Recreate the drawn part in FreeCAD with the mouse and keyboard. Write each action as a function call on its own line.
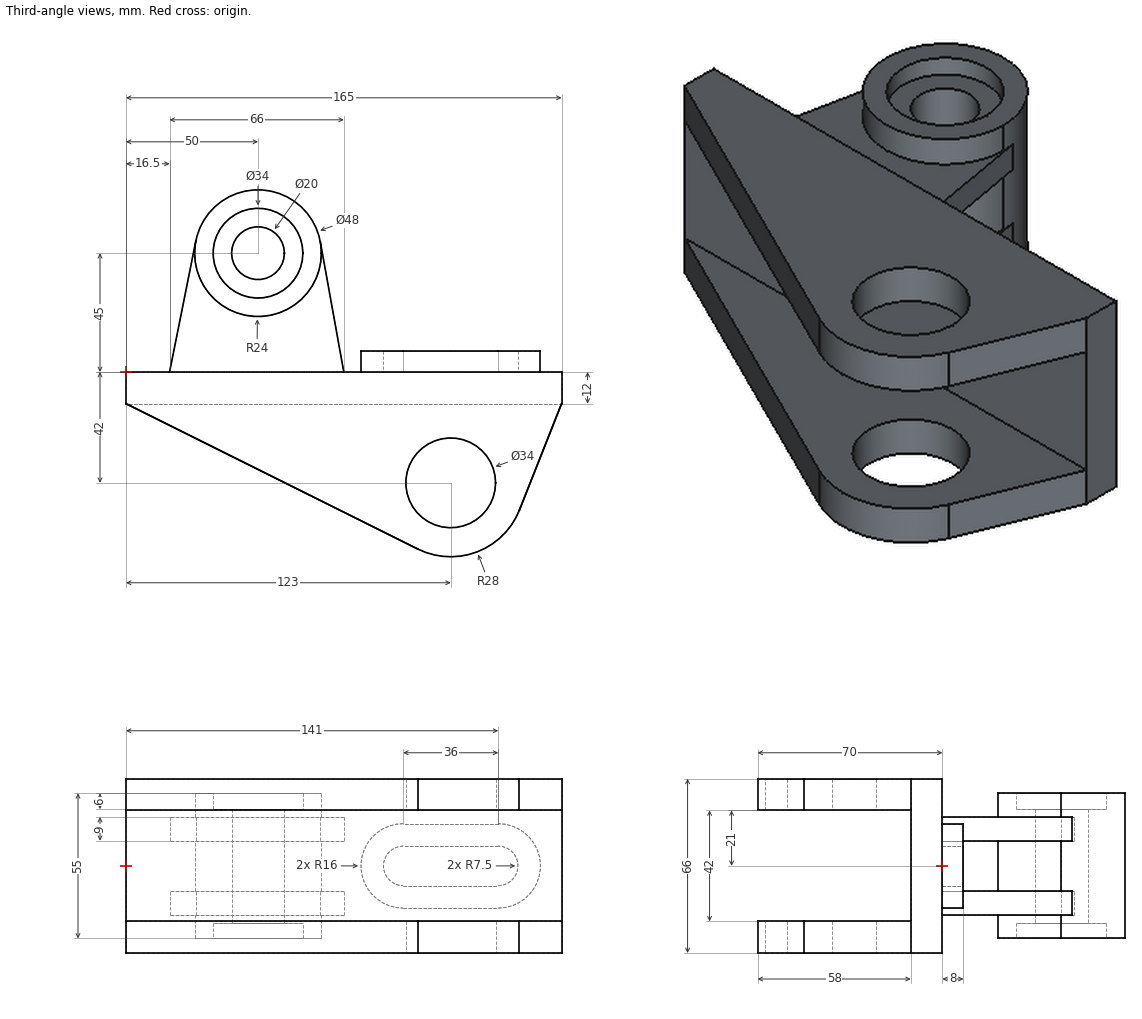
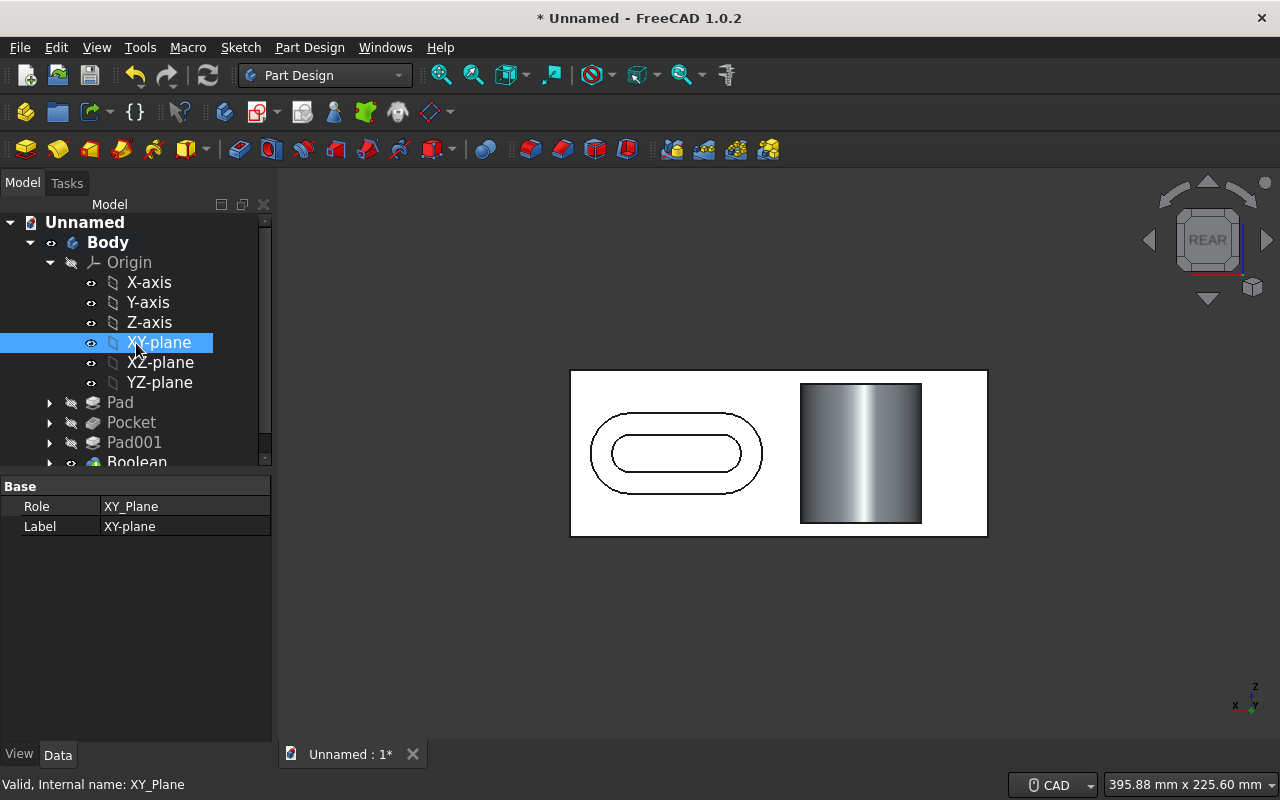
click(430, 112)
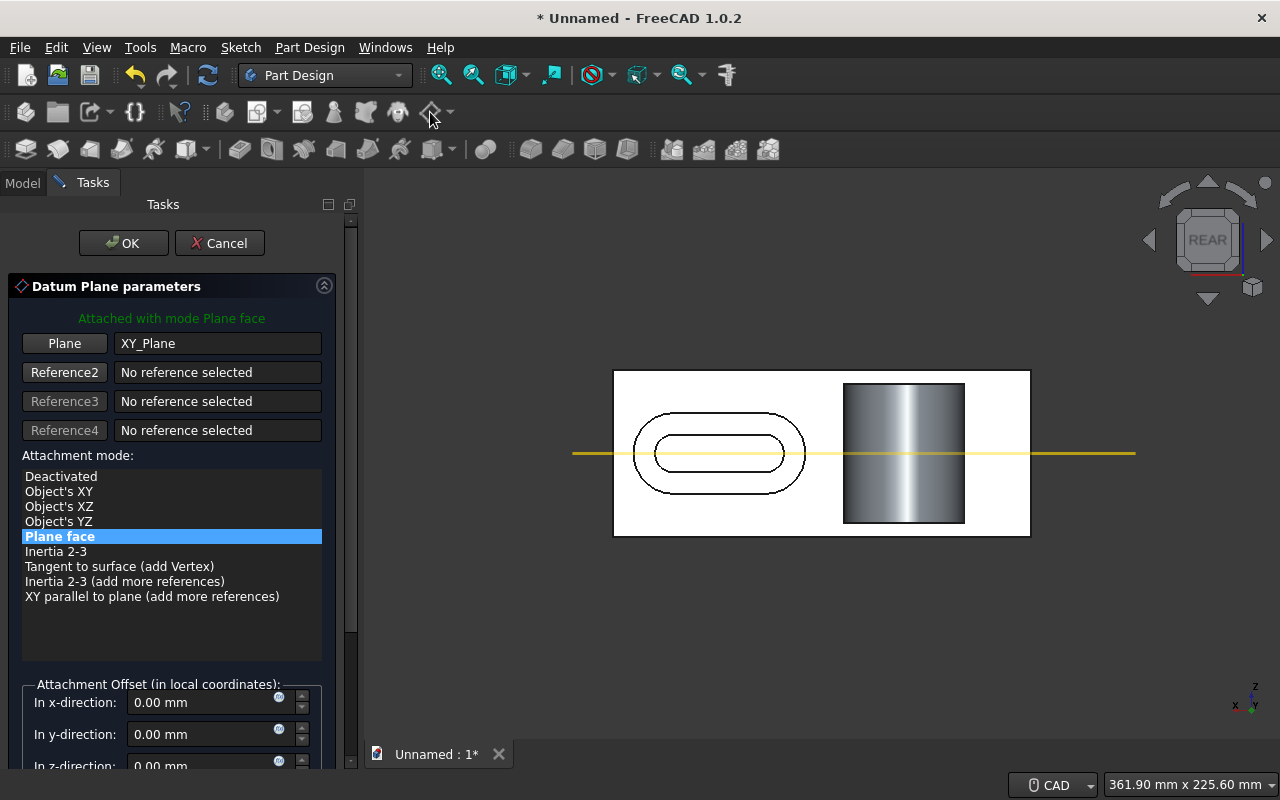
scroll(351, 491, down, 2)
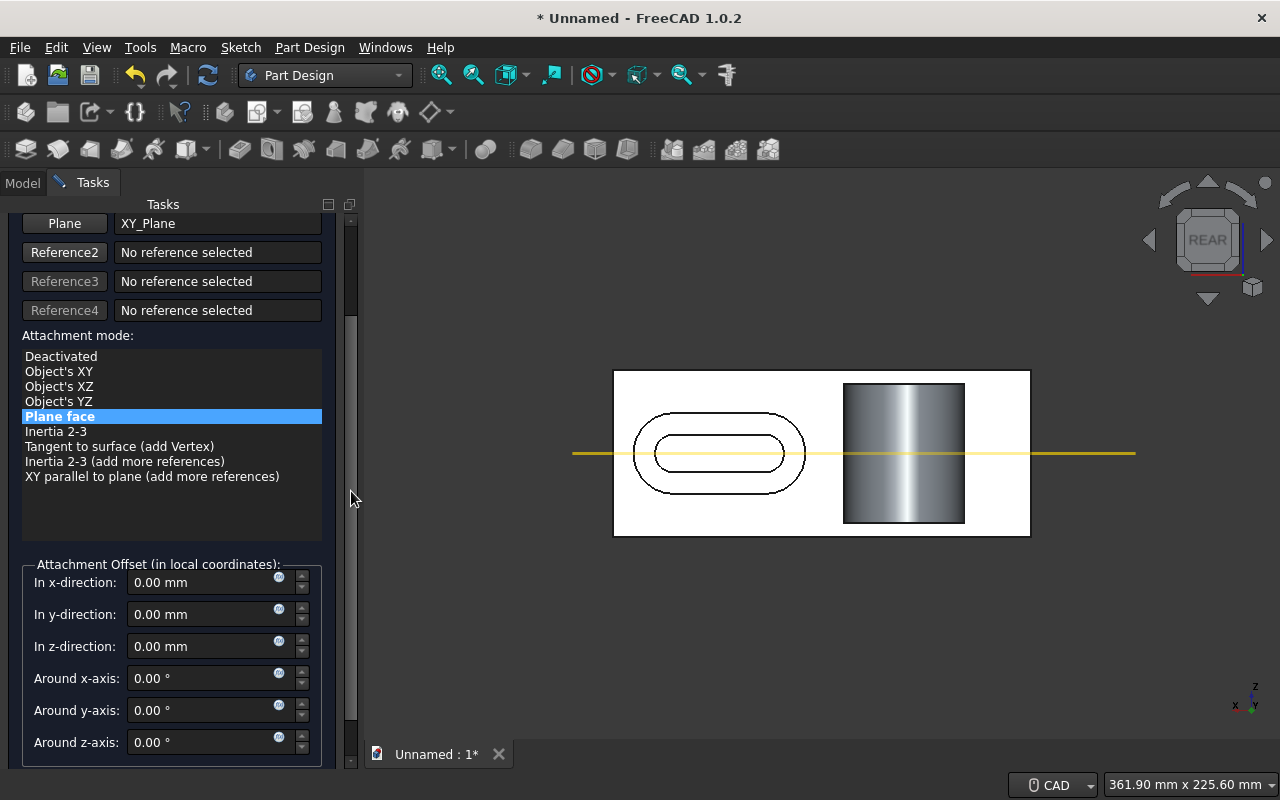
triple_click(210, 646)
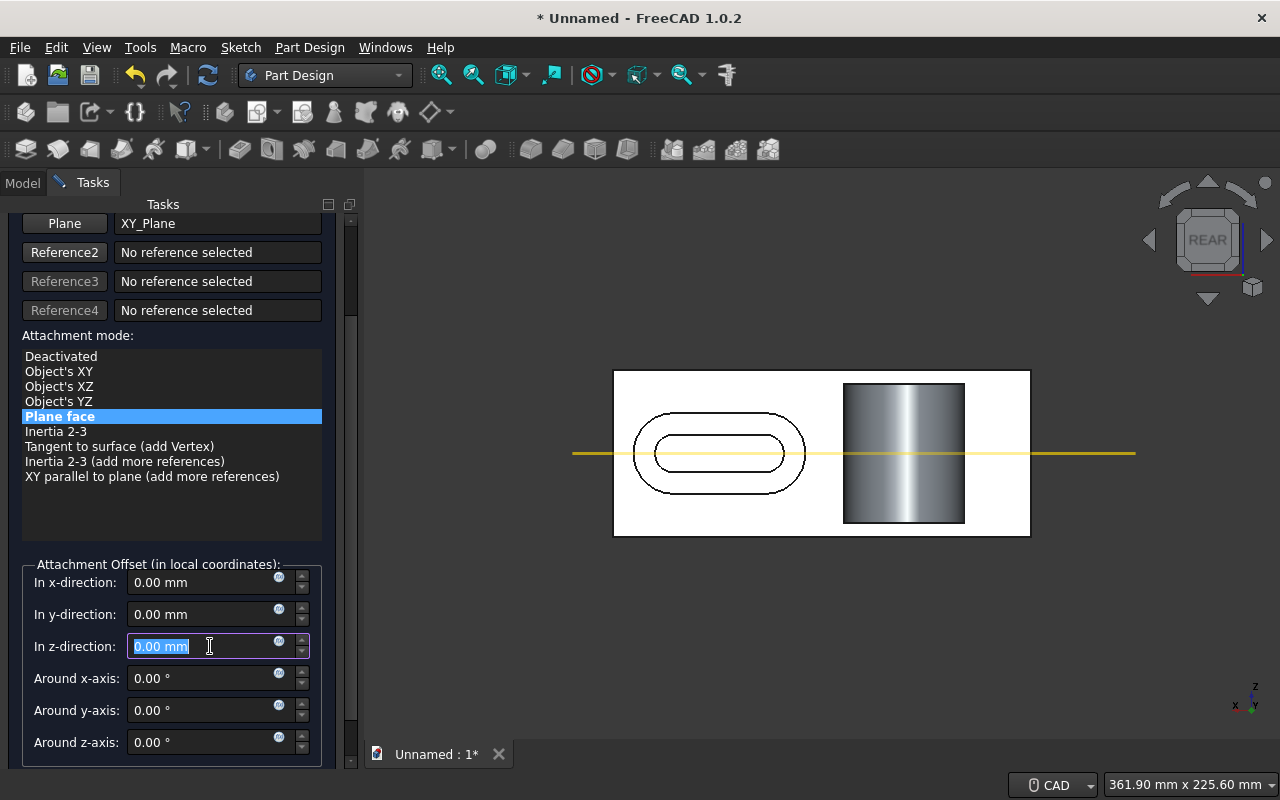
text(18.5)
key(Tab)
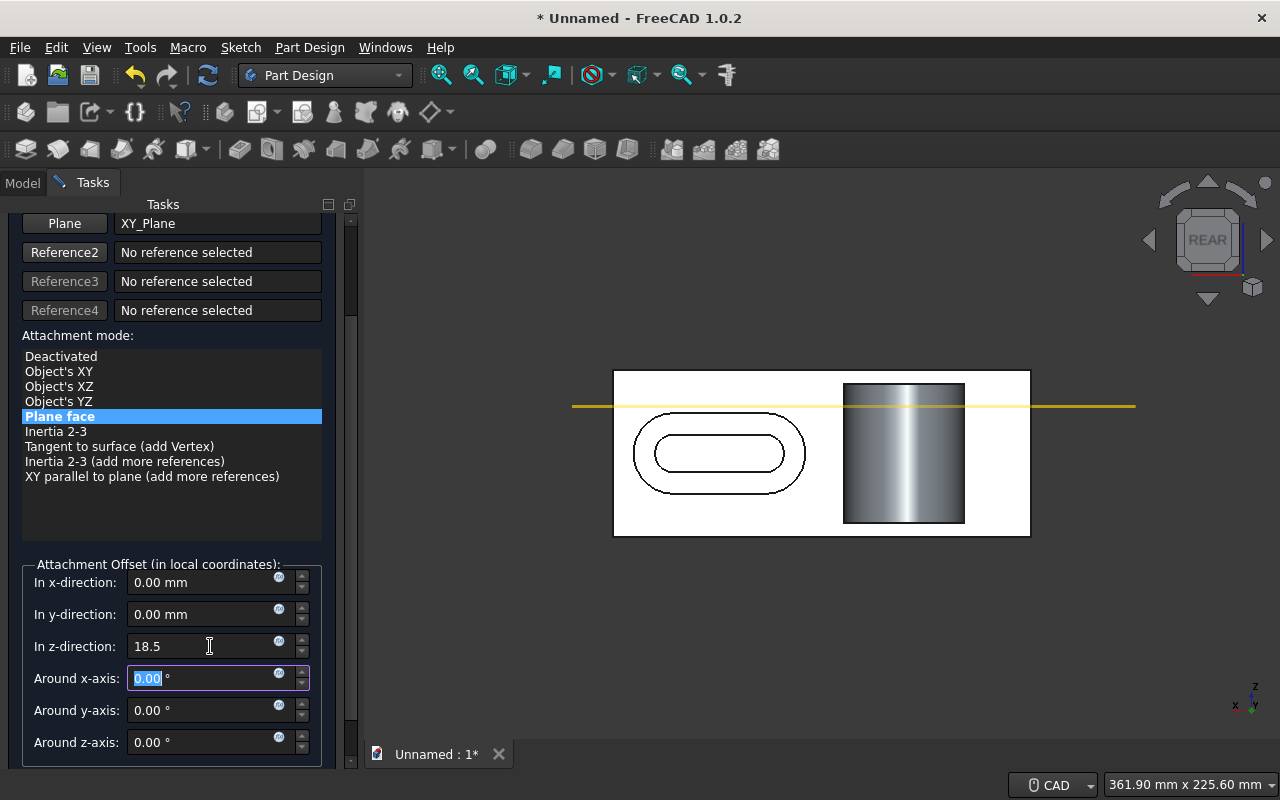
scroll(351, 491, up, 3)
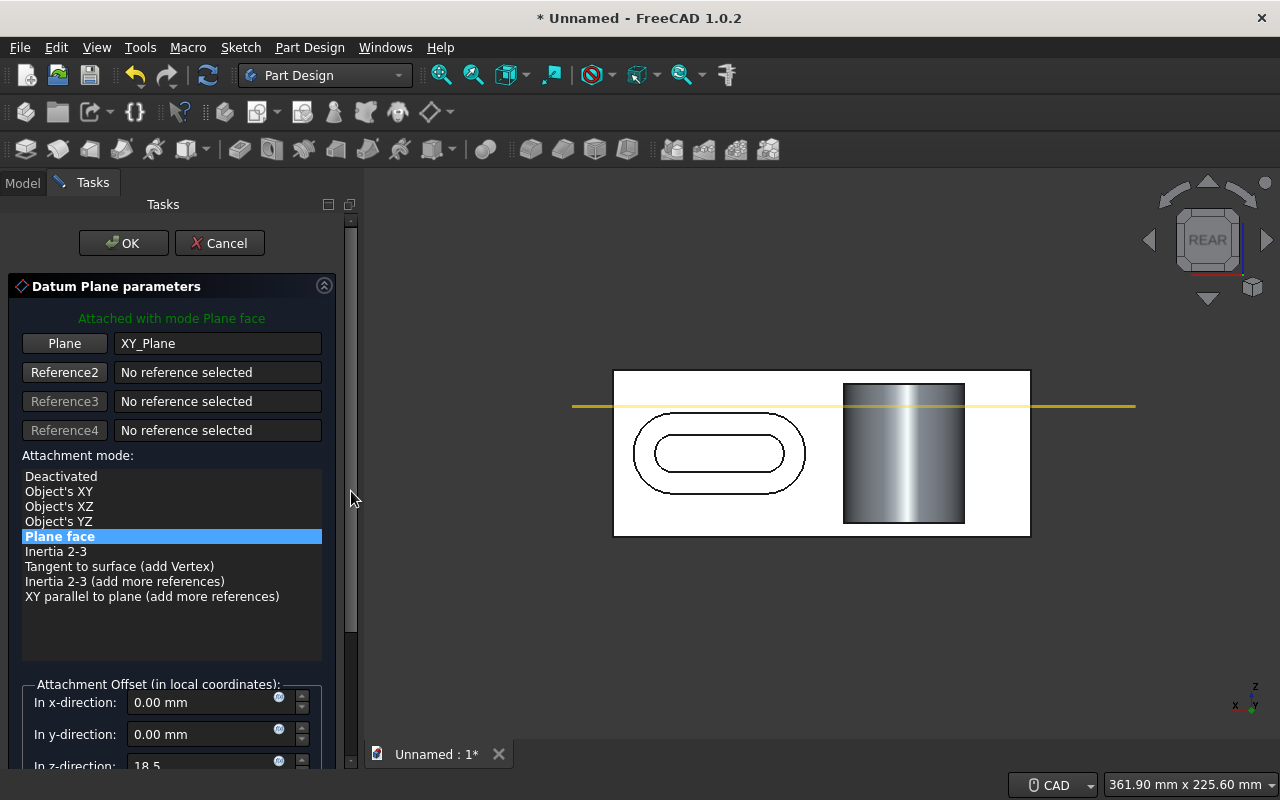
click(124, 243)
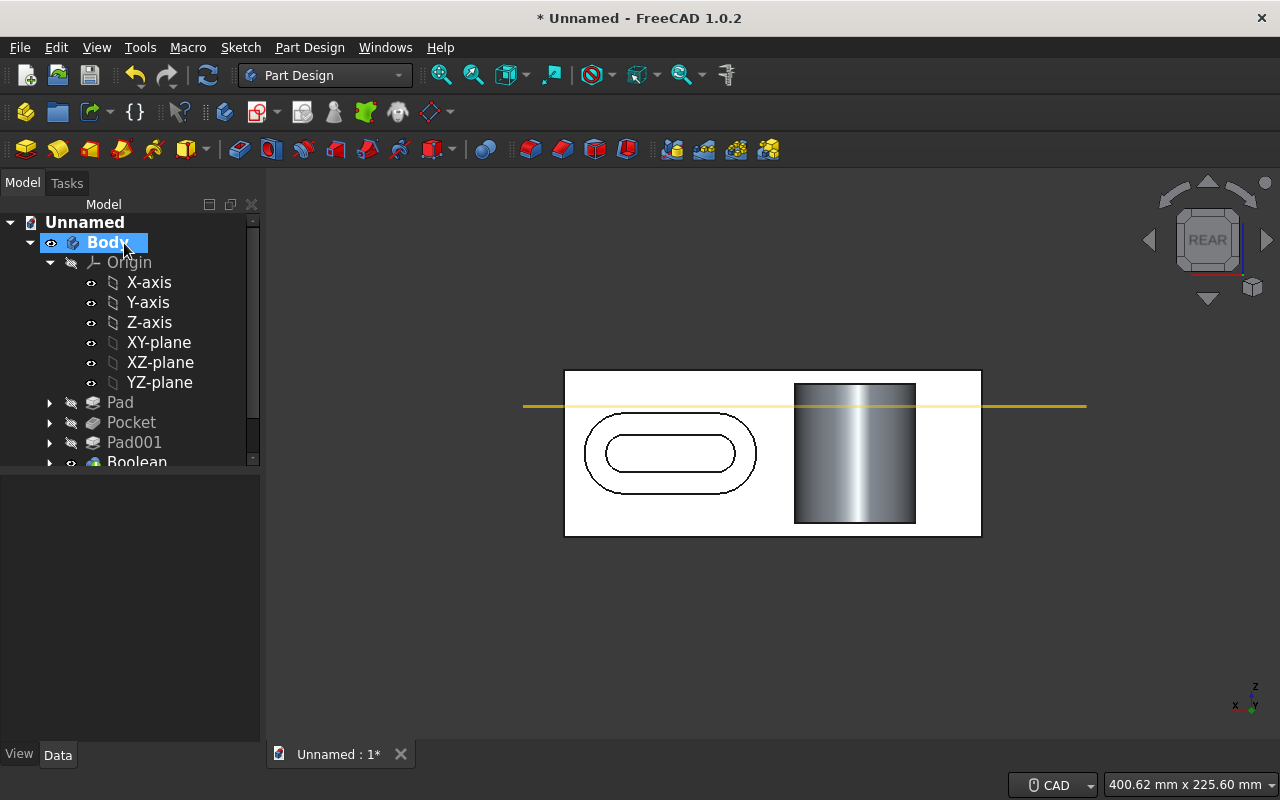
scroll(100, 338, down, 3)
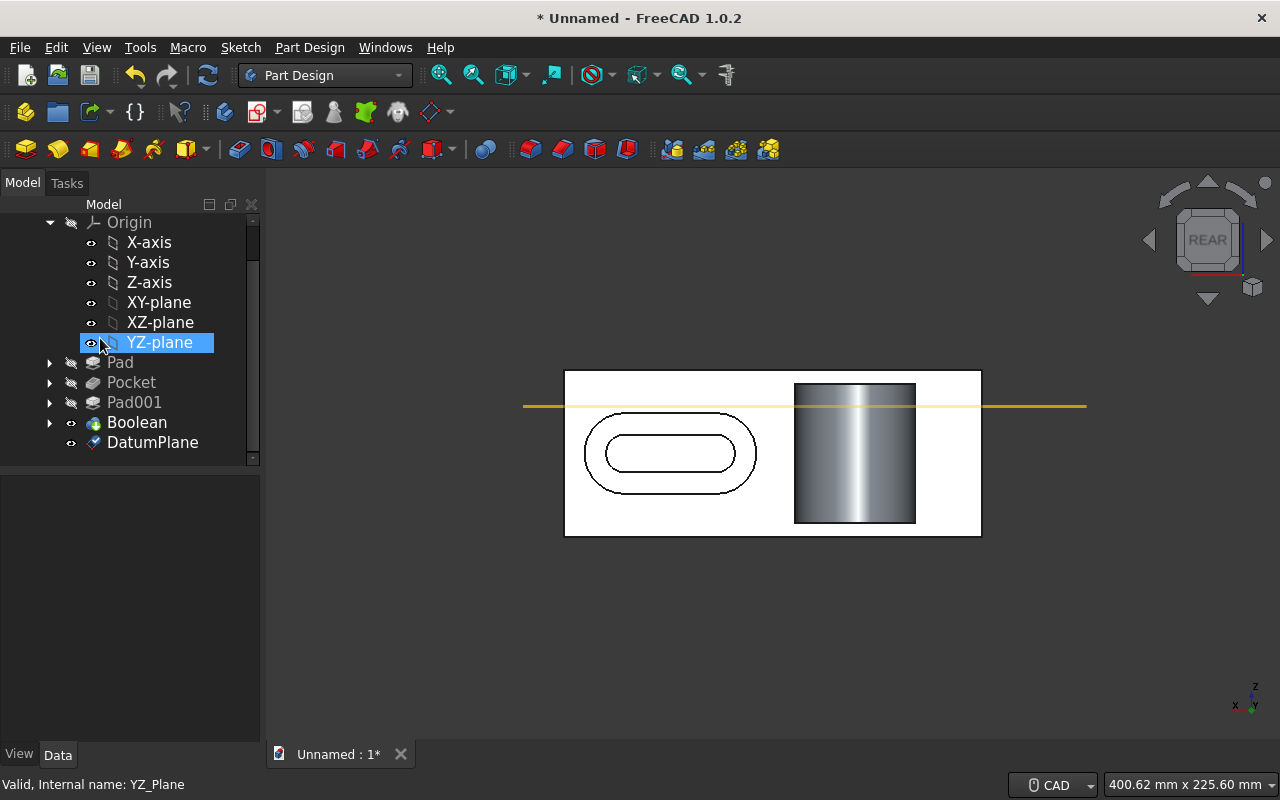
click(116, 443)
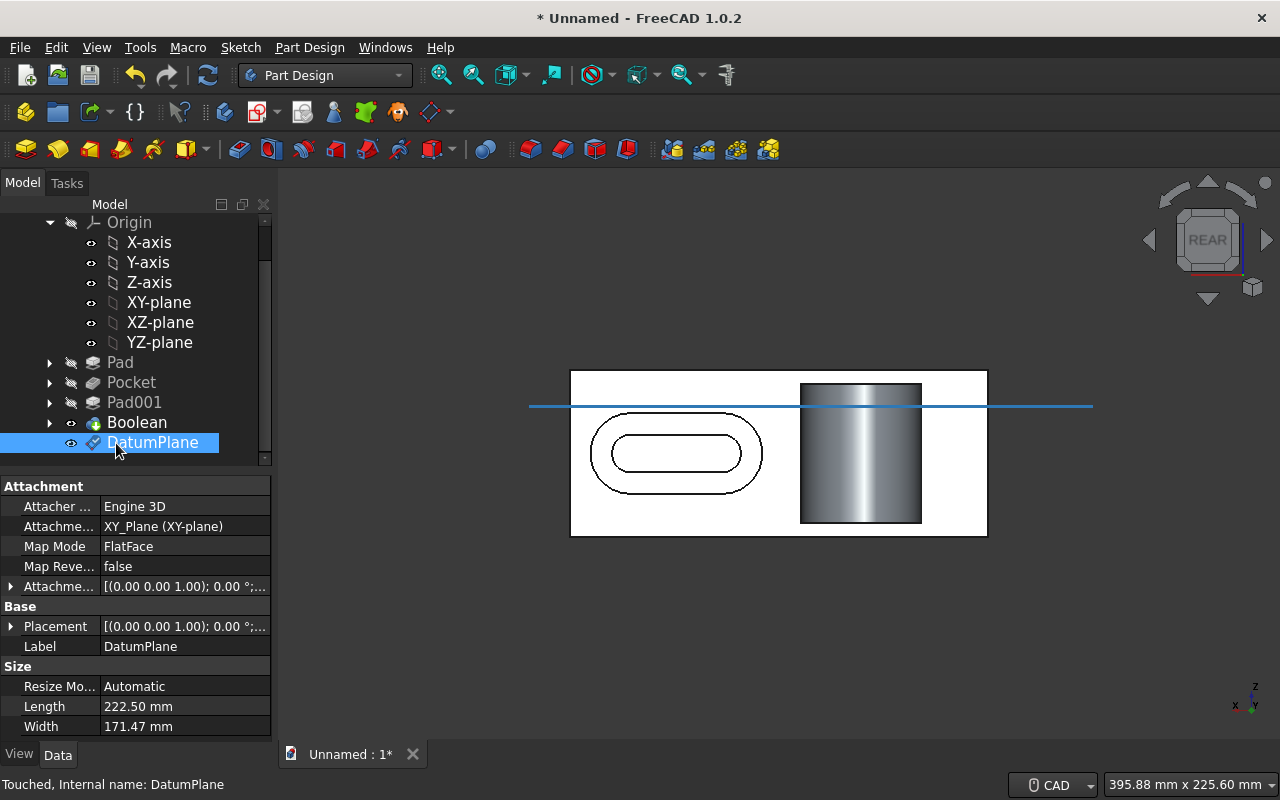
click(258, 112)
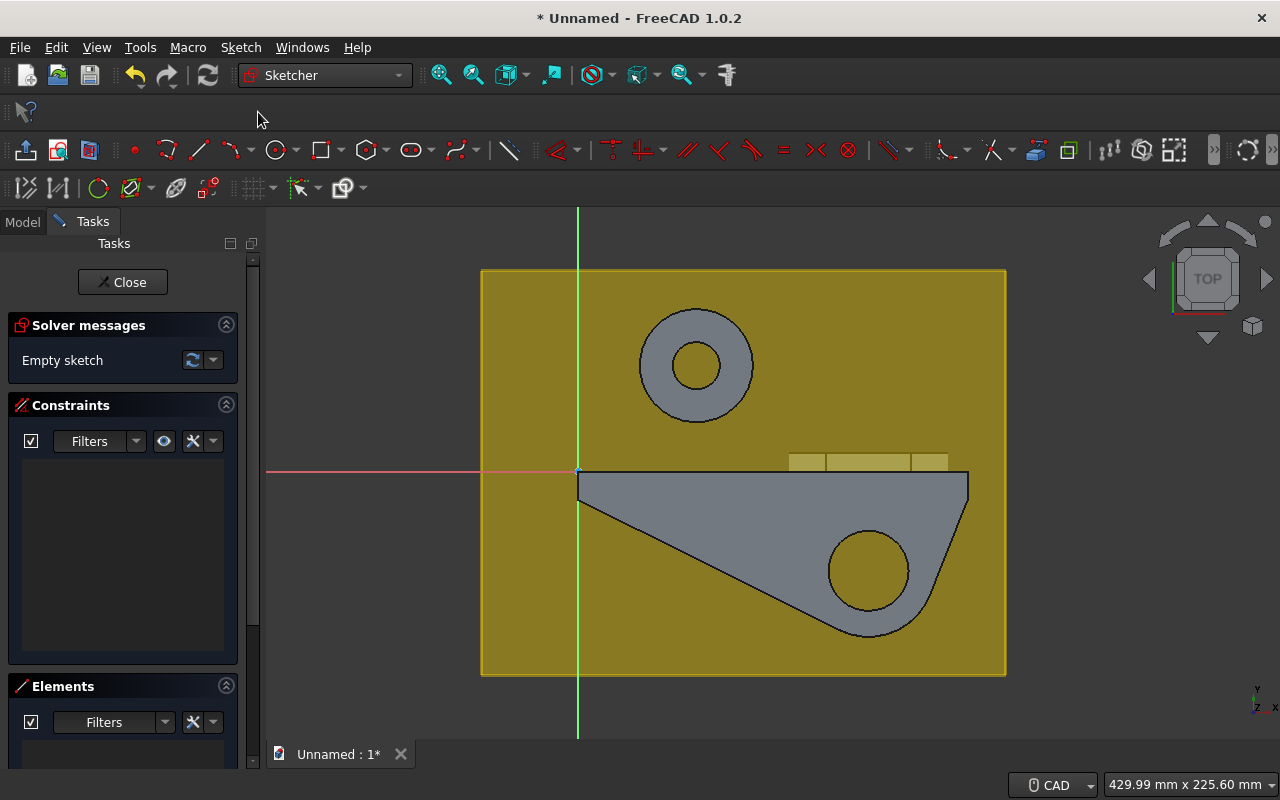
key(q)
key(s)